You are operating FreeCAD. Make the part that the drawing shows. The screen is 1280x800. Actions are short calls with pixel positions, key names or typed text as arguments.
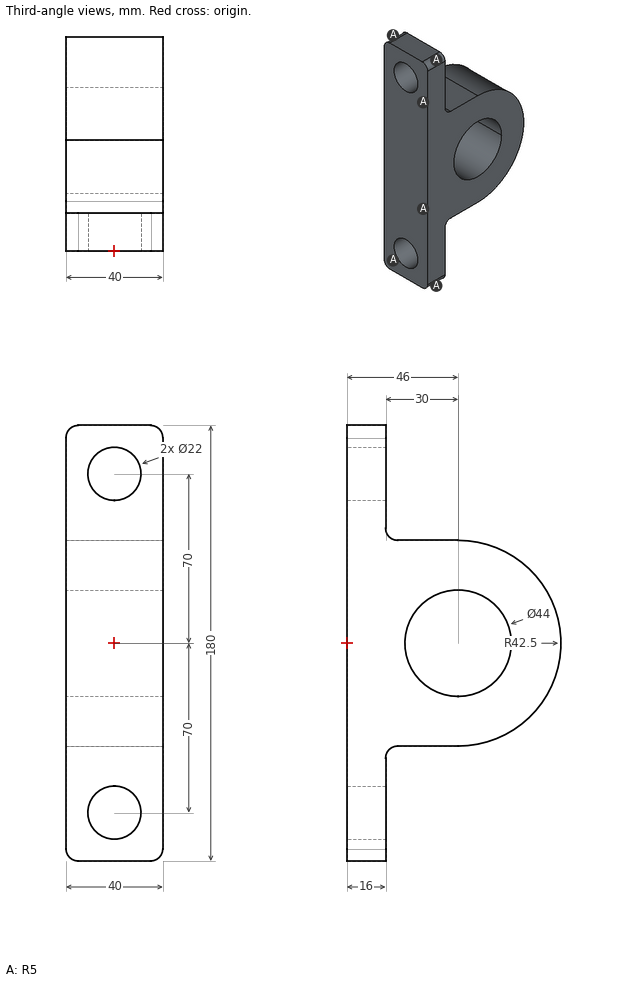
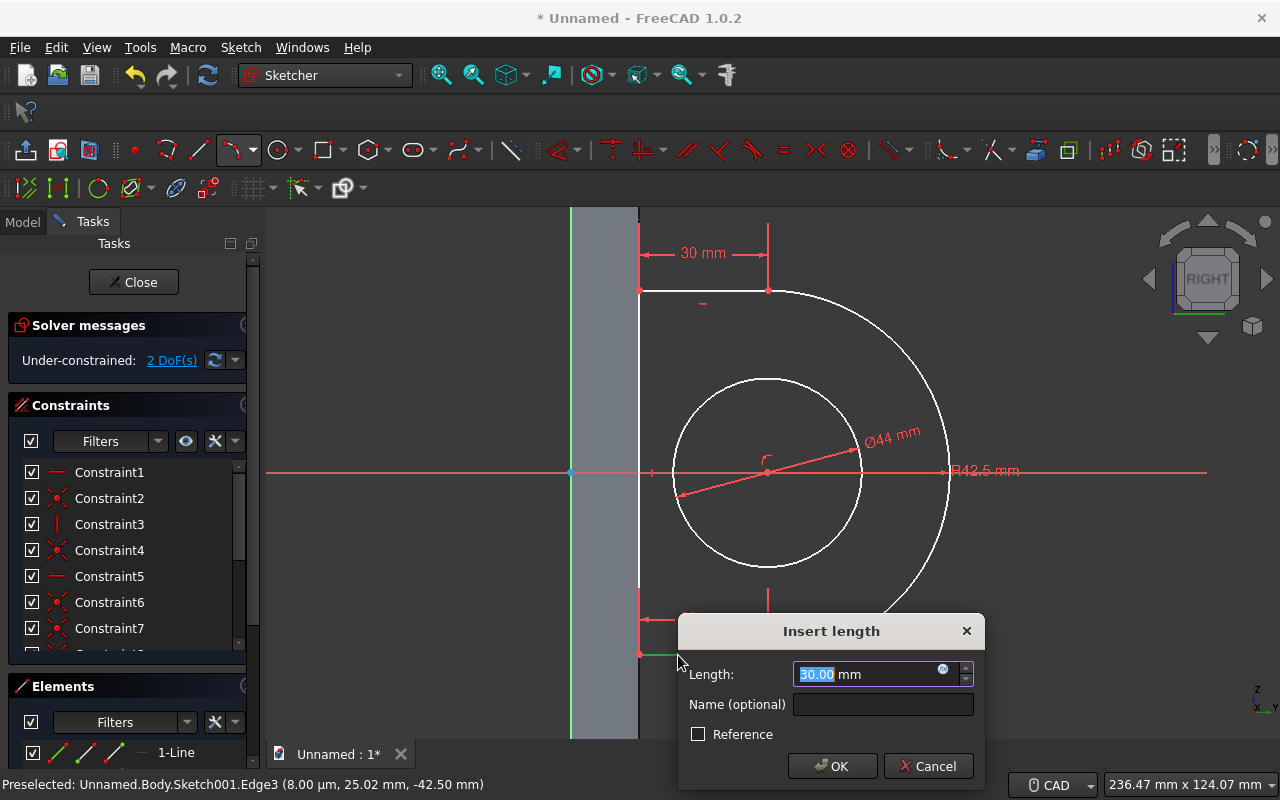
text(30)
key(Return)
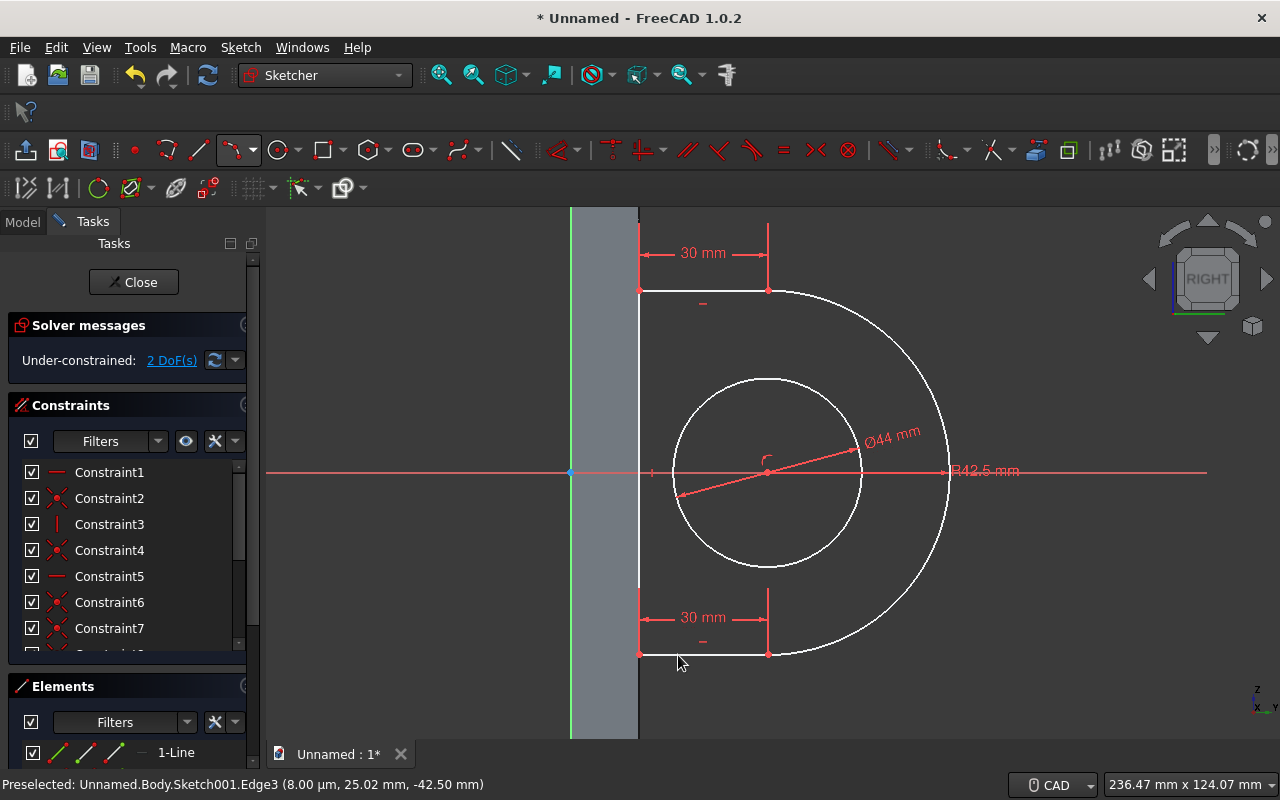
click(767, 473)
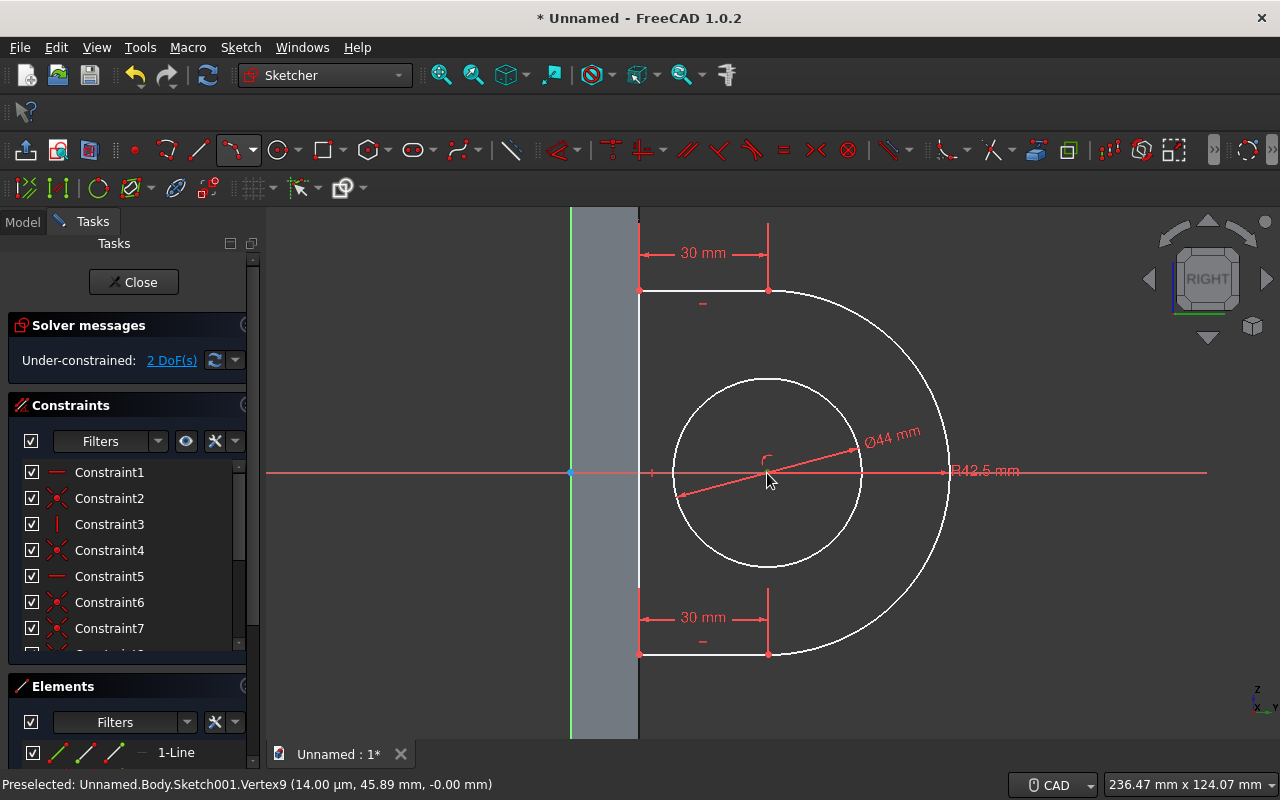
key(l)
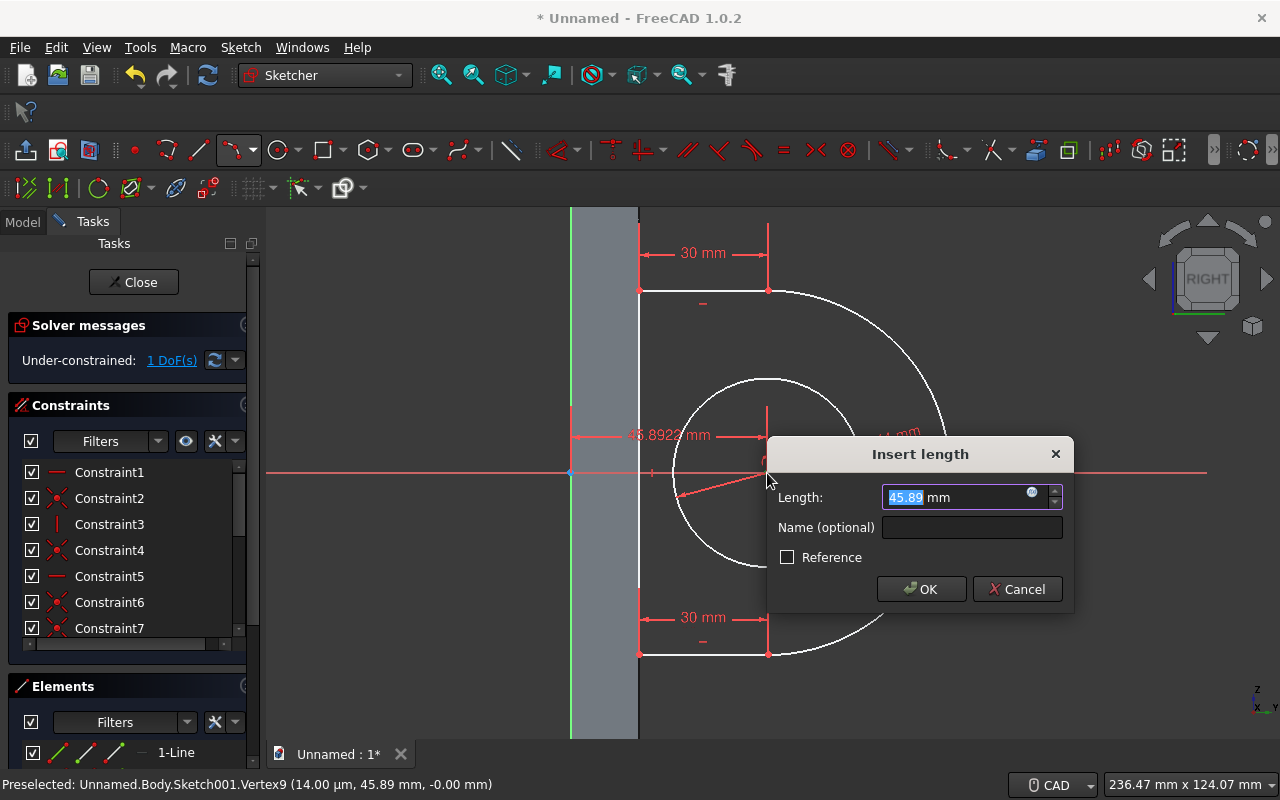
text(46)
key(Return)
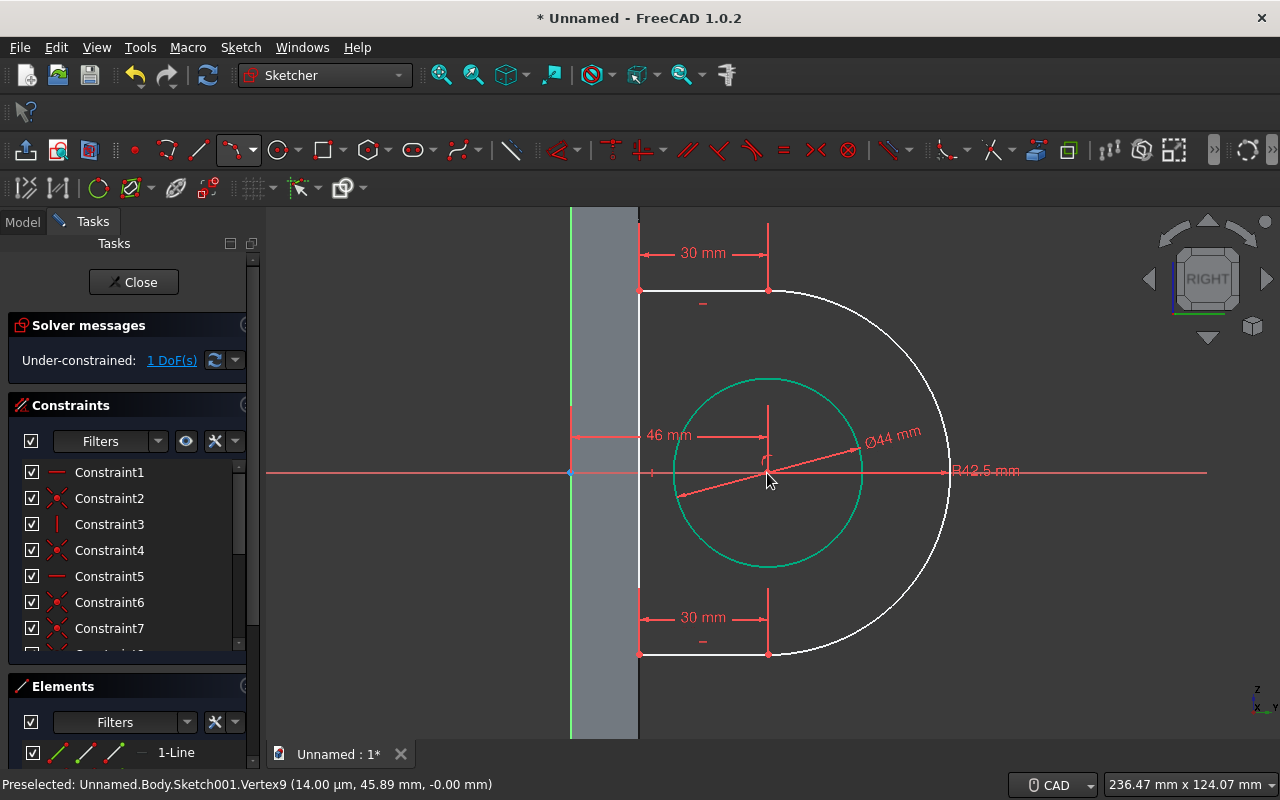
click(768, 291)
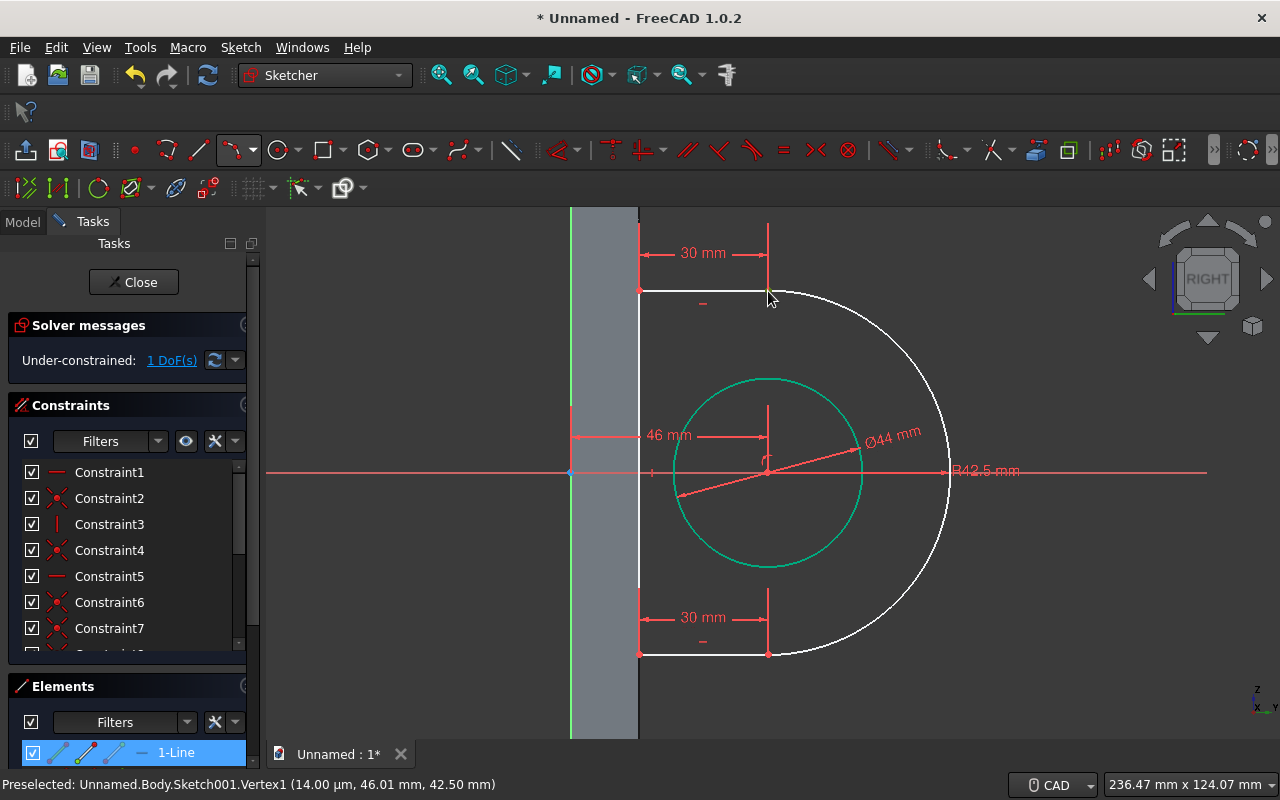
click(580, 150)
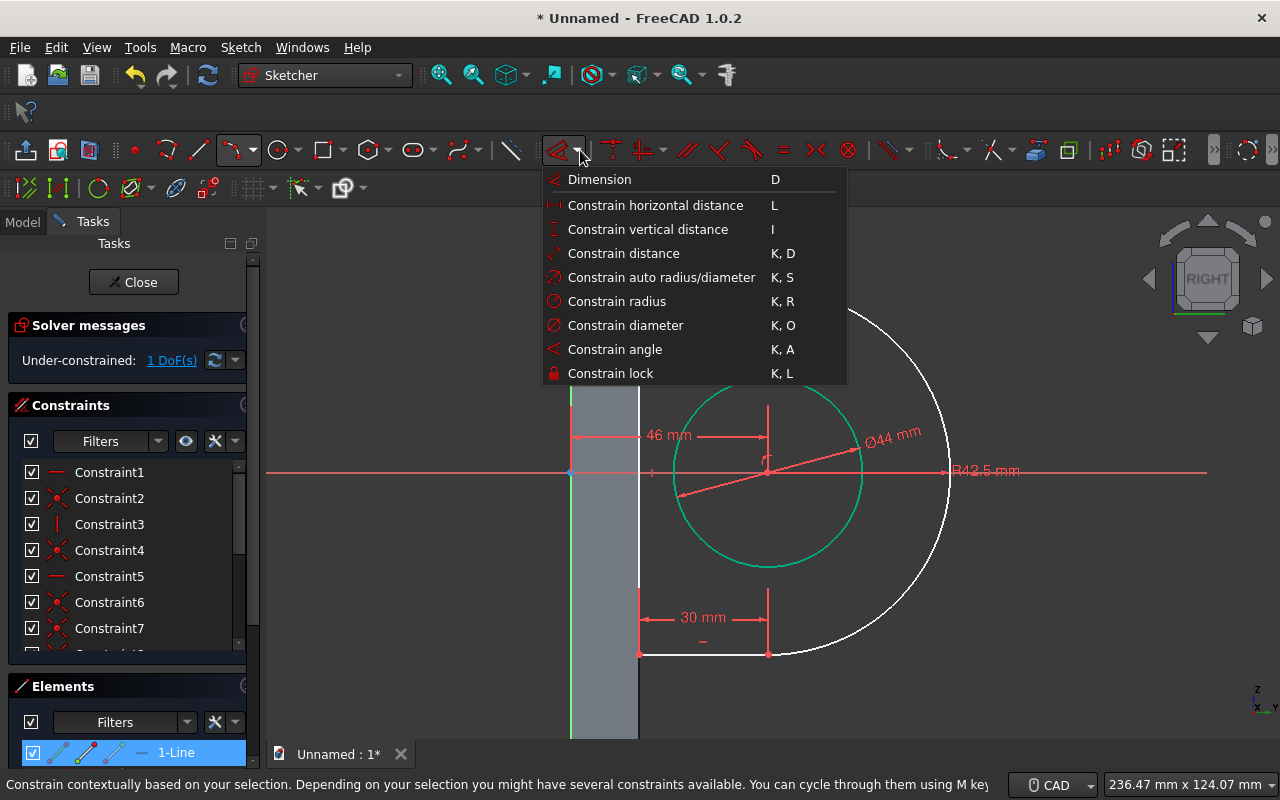
click(695, 205)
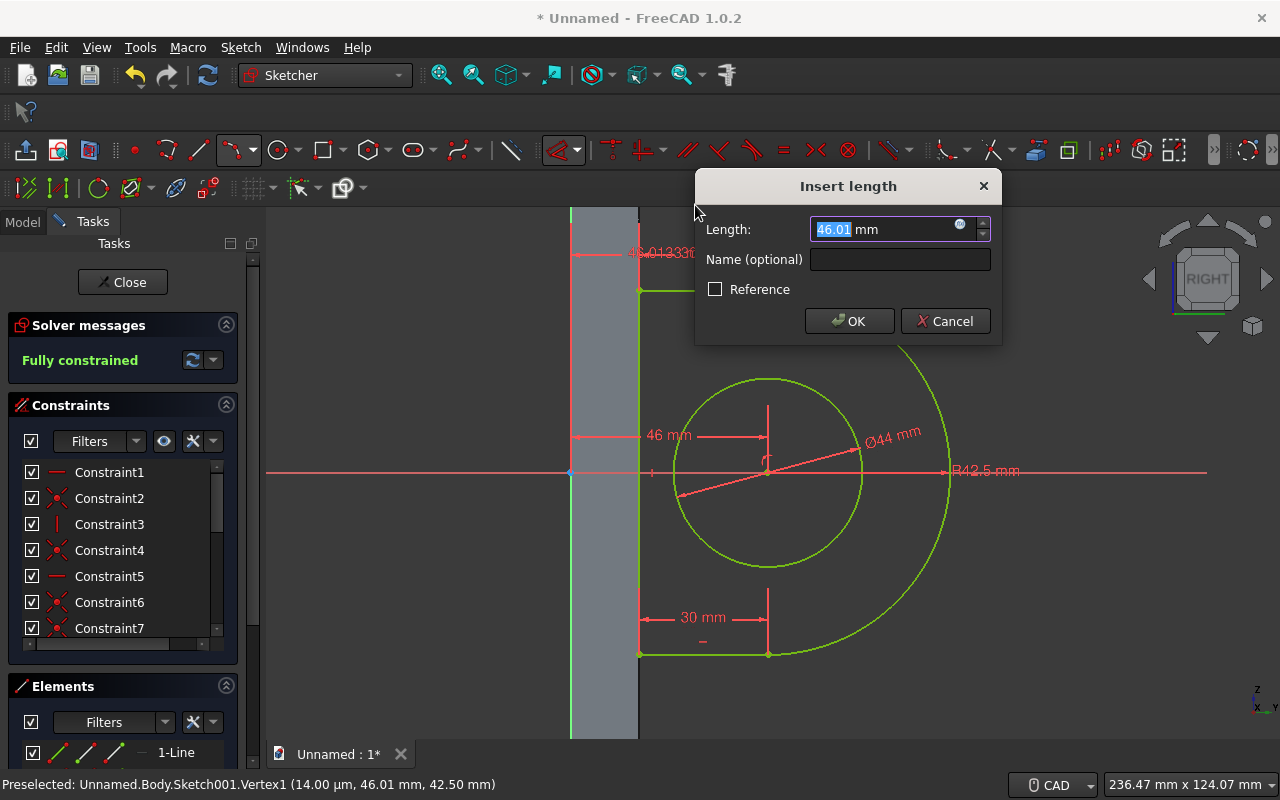
text(46)
key(Return)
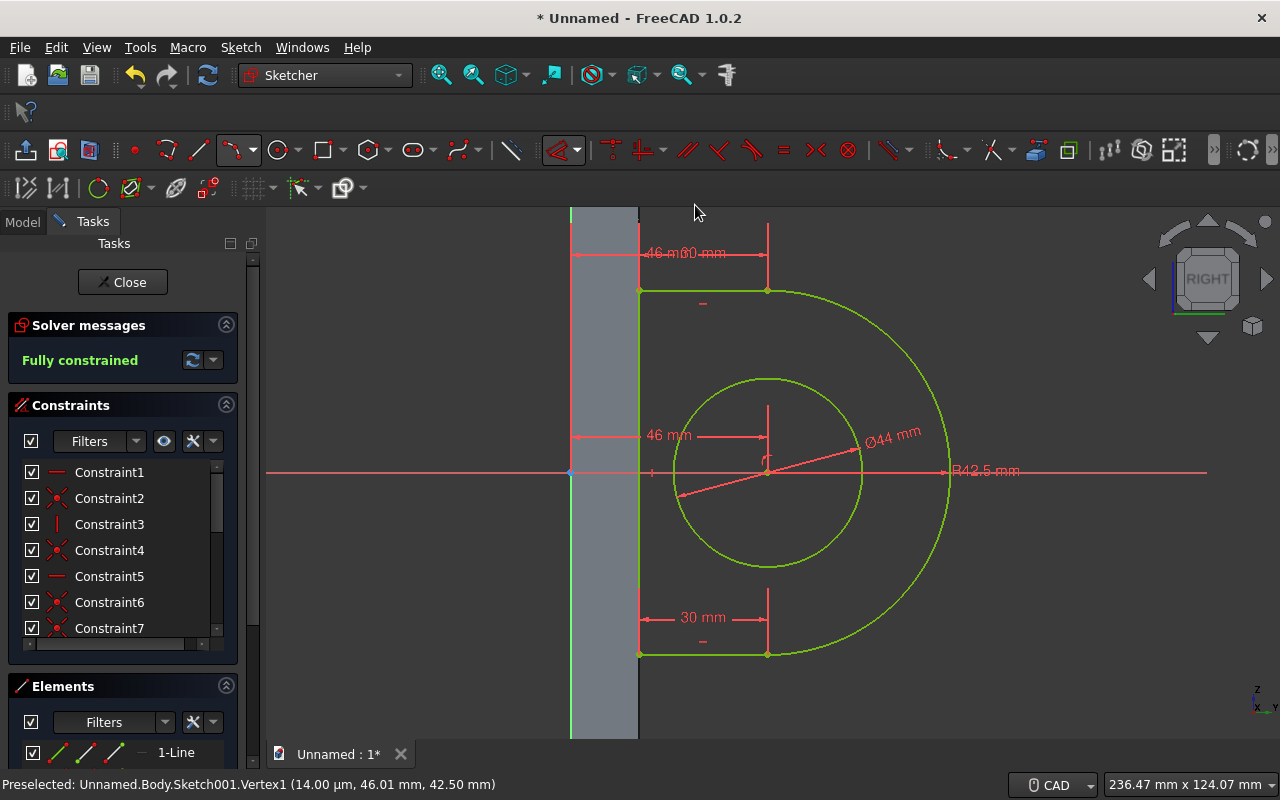
click(123, 282)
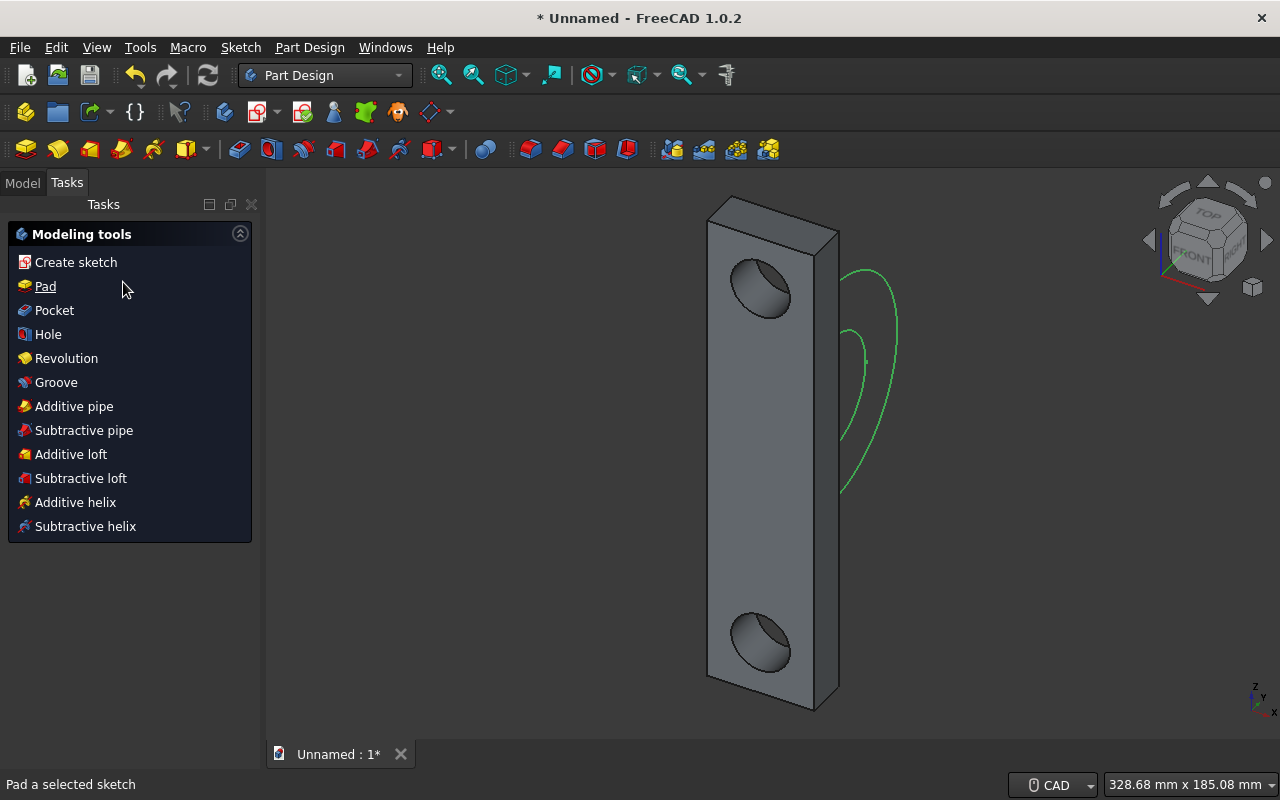
click(26, 150)